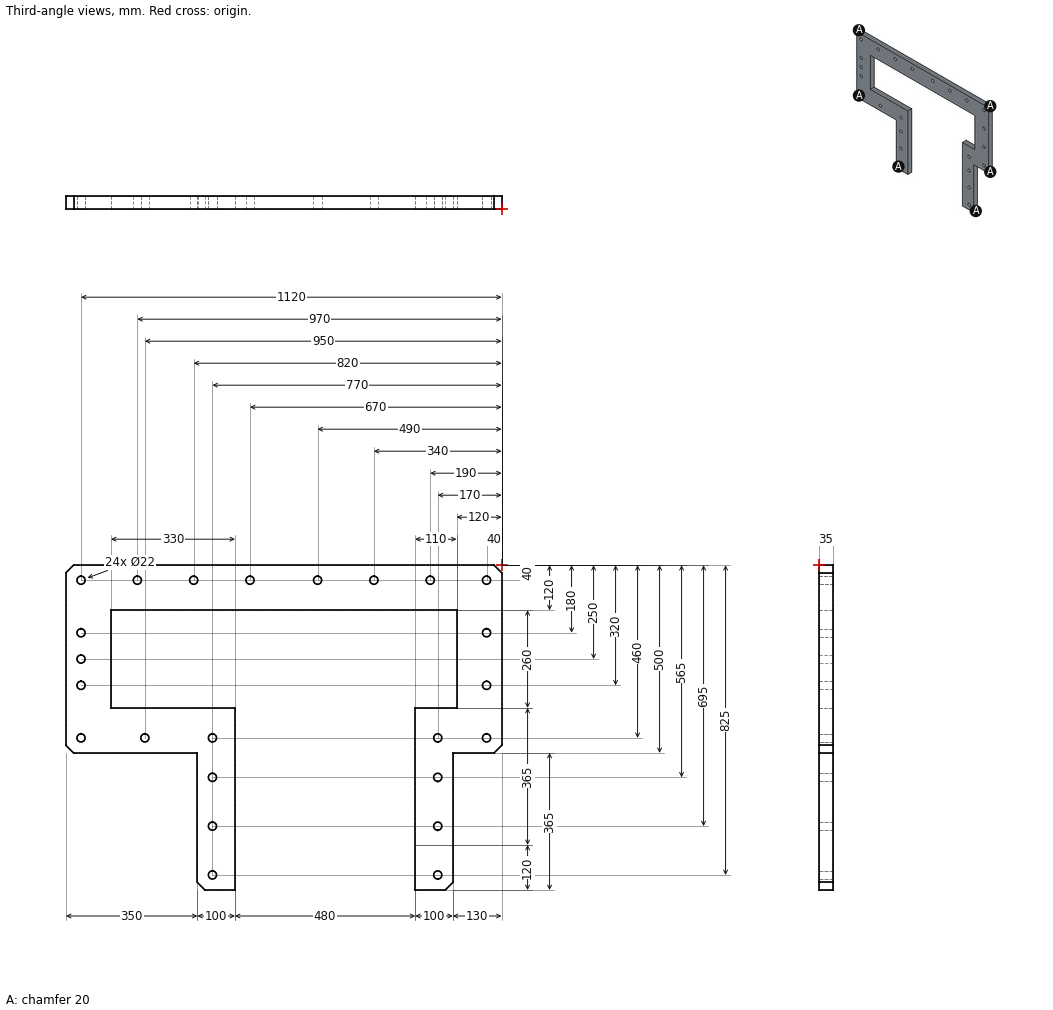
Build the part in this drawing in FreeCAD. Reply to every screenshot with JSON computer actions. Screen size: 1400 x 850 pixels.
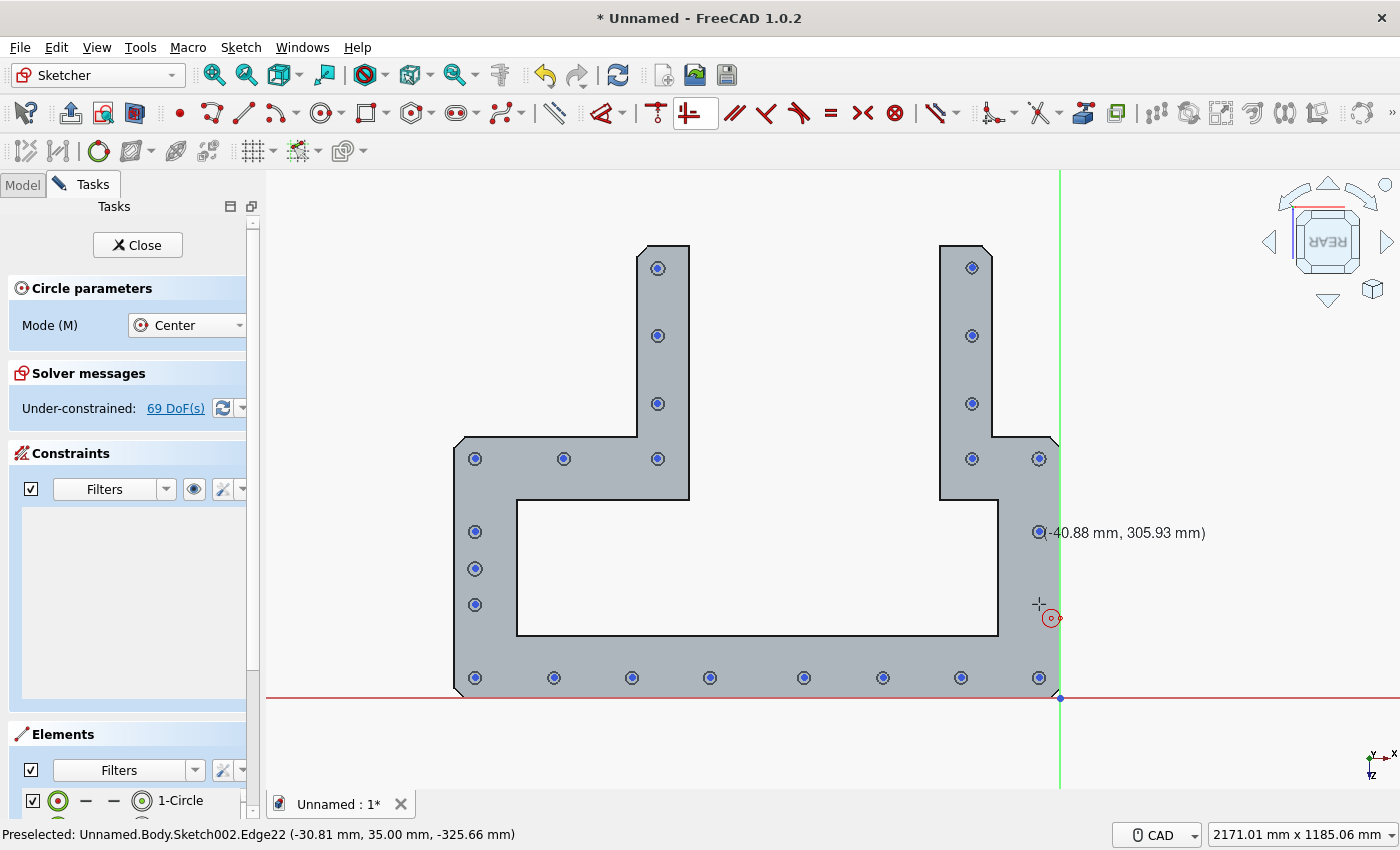
{"action": "left_click", "coordinate": [1039, 604]}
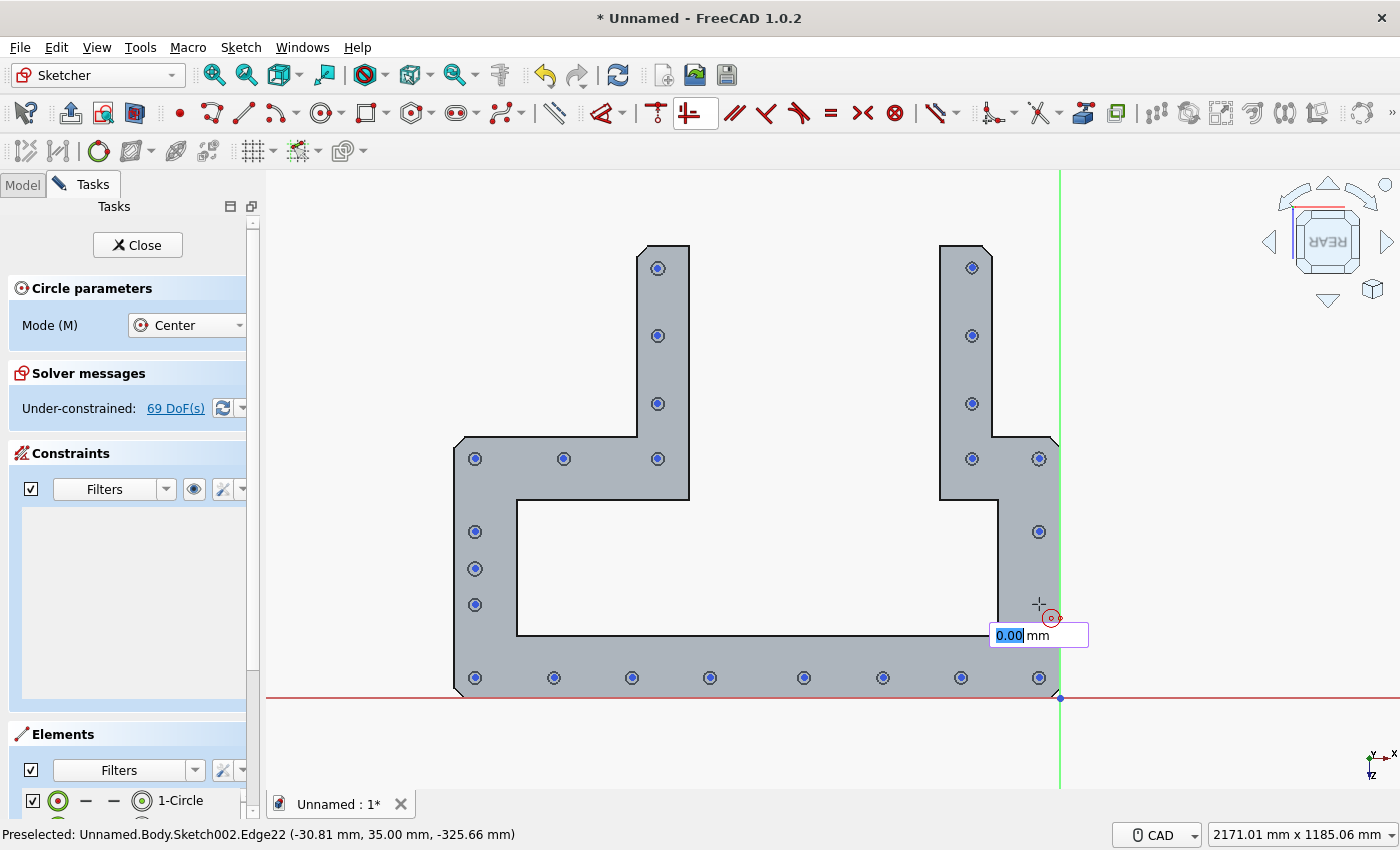
{"action": "scroll", "coordinate": [1044, 600], "scroll_direction": "up", "scroll_amount": 6}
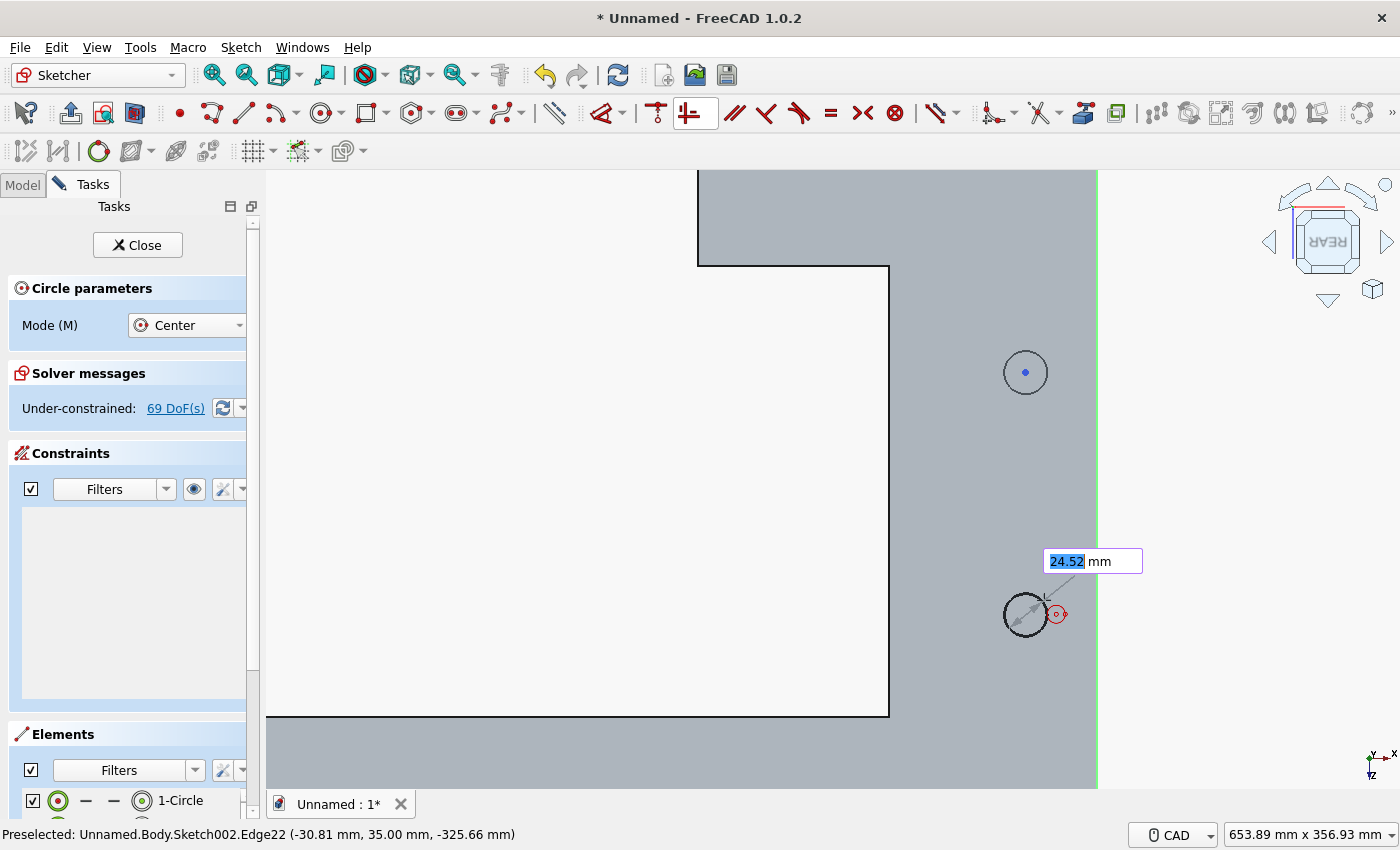
{"action": "left_click", "coordinate": [1041, 599]}
{"action": "key", "text": "Escape"}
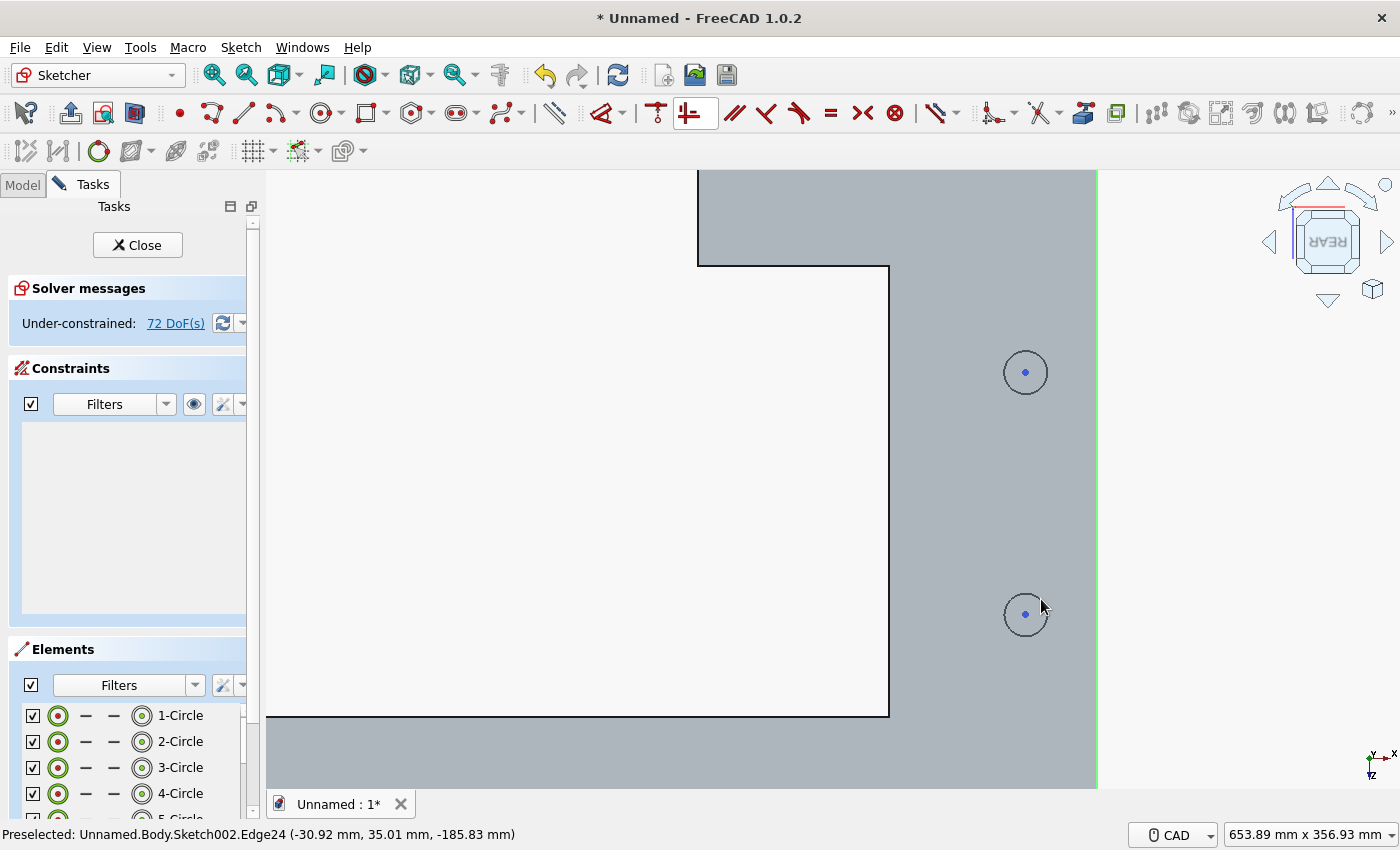
{"action": "scroll", "coordinate": [1044, 600], "scroll_direction": "down", "scroll_amount": 6}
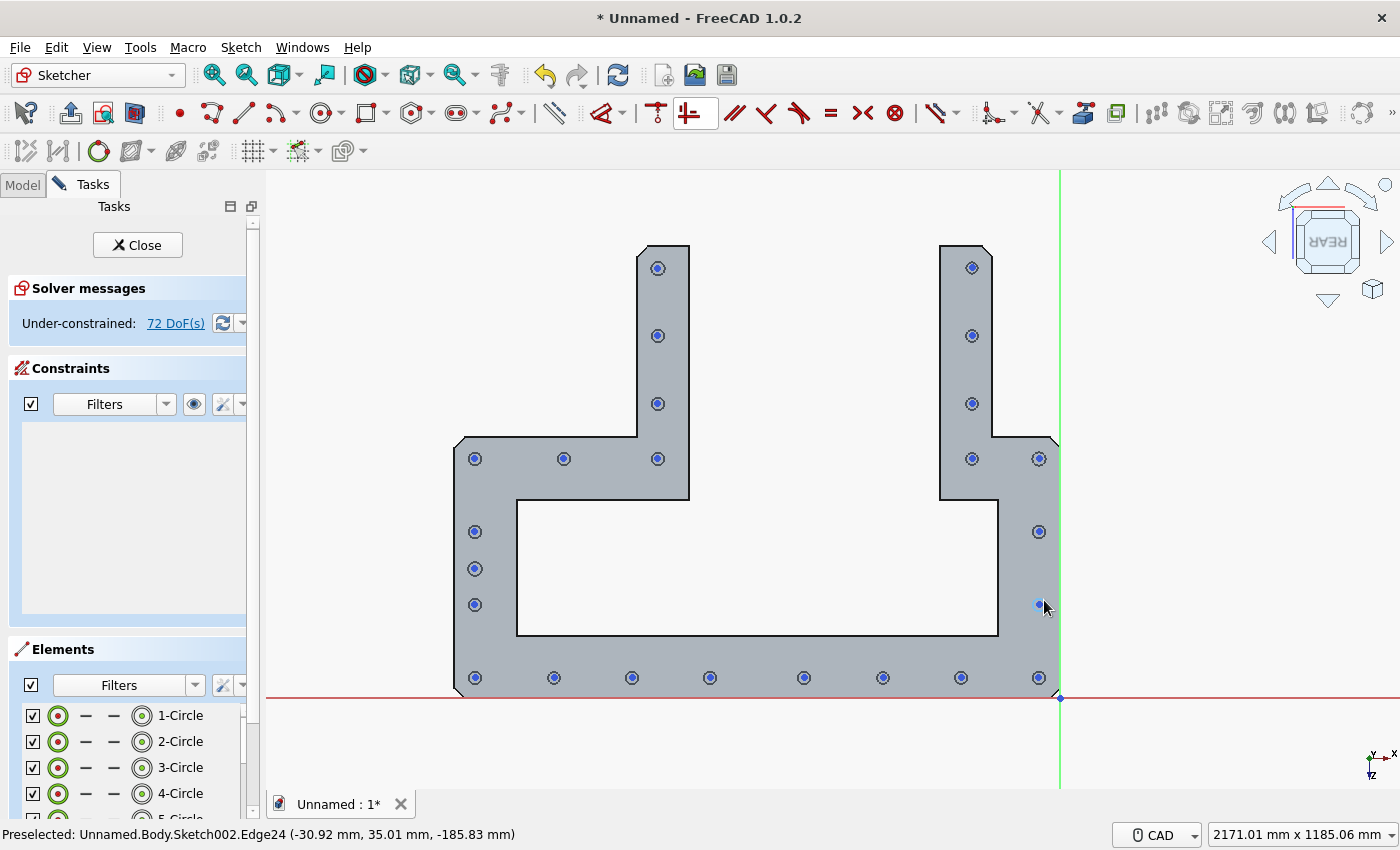
{"action": "scroll", "coordinate": [479, 673], "scroll_direction": "up", "scroll_amount": 4}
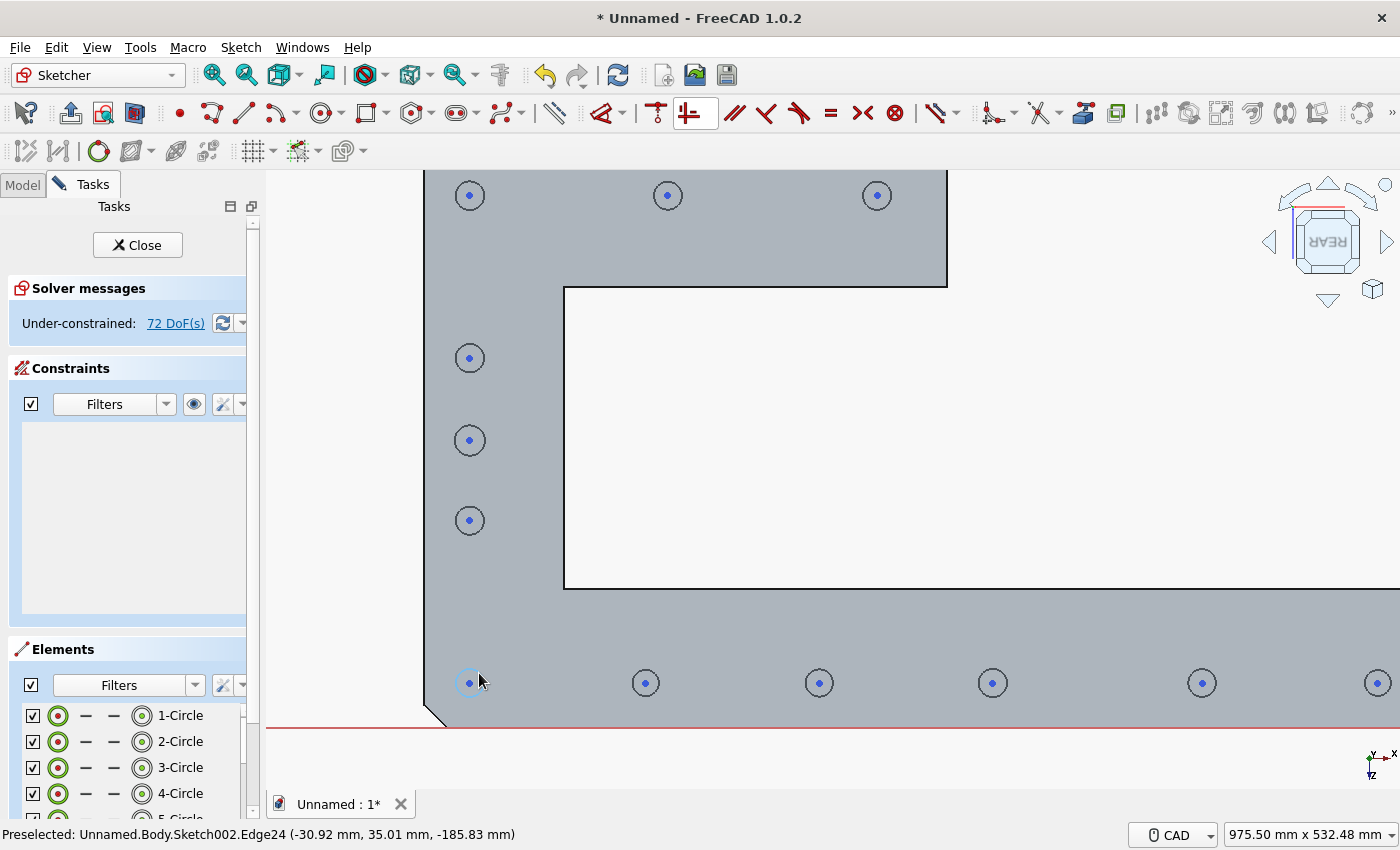
{"action": "left_click", "coordinate": [480, 673]}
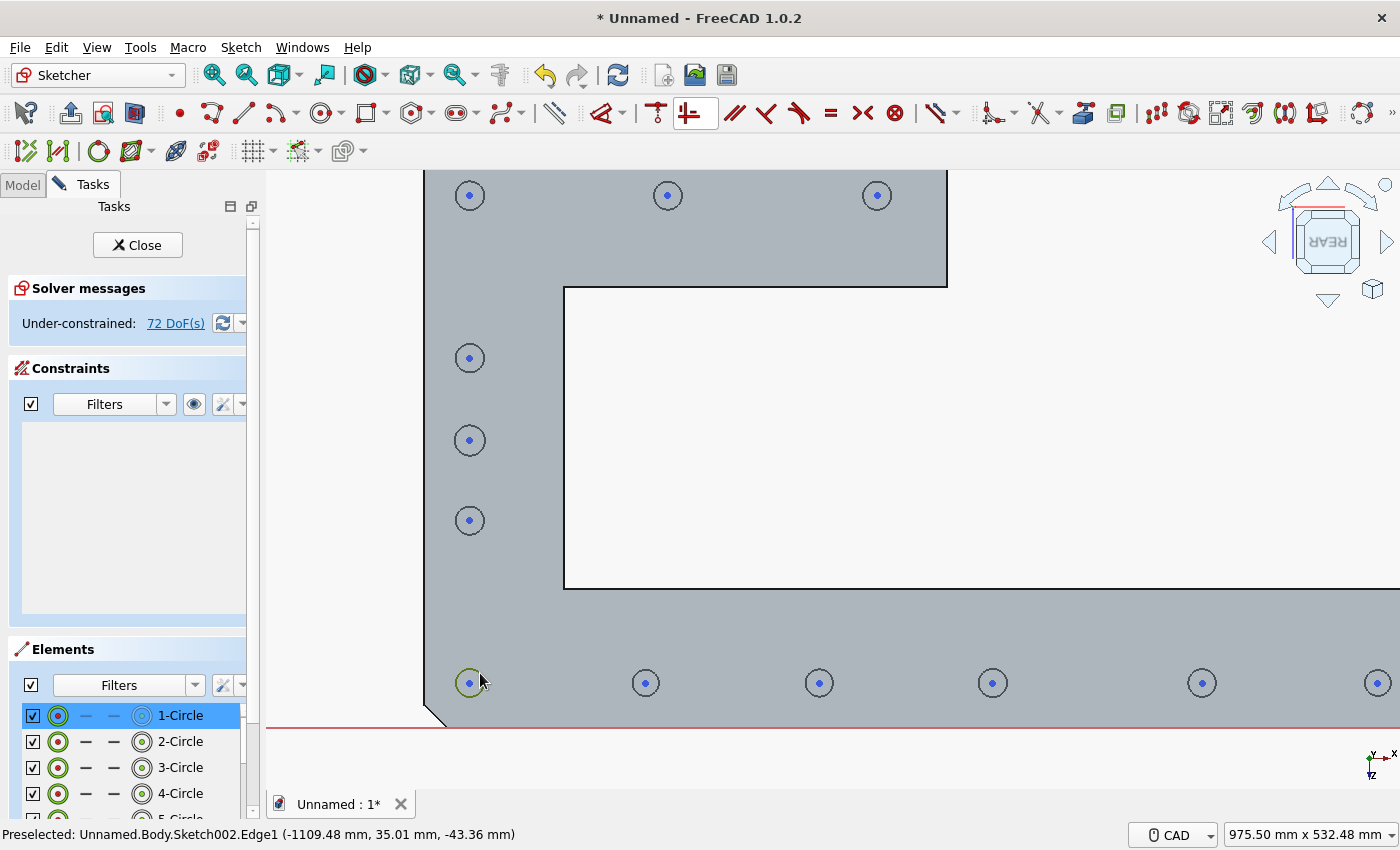
{"action": "left_click", "coordinate": [655, 674]}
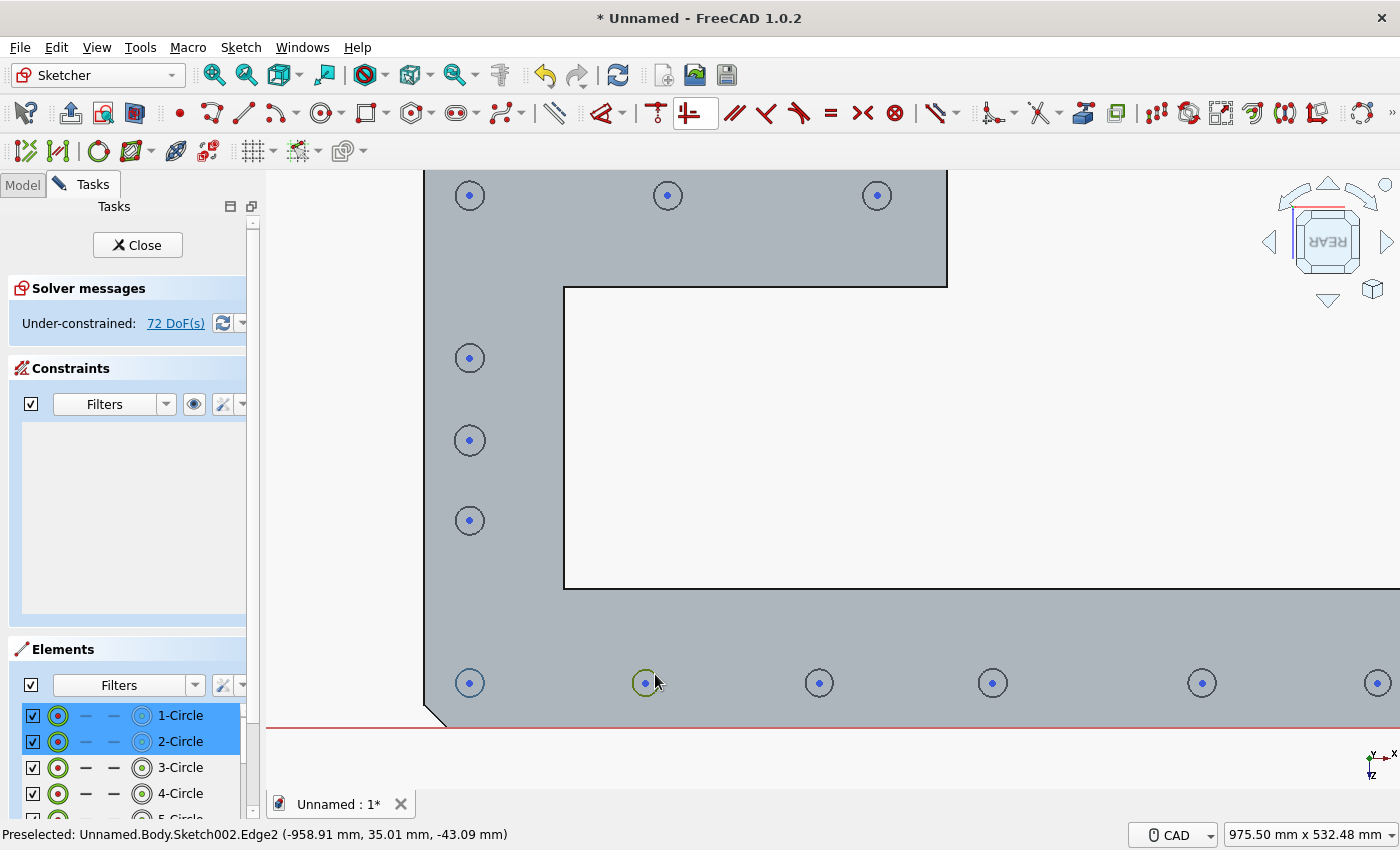
{"action": "left_click", "coordinate": [829, 673]}